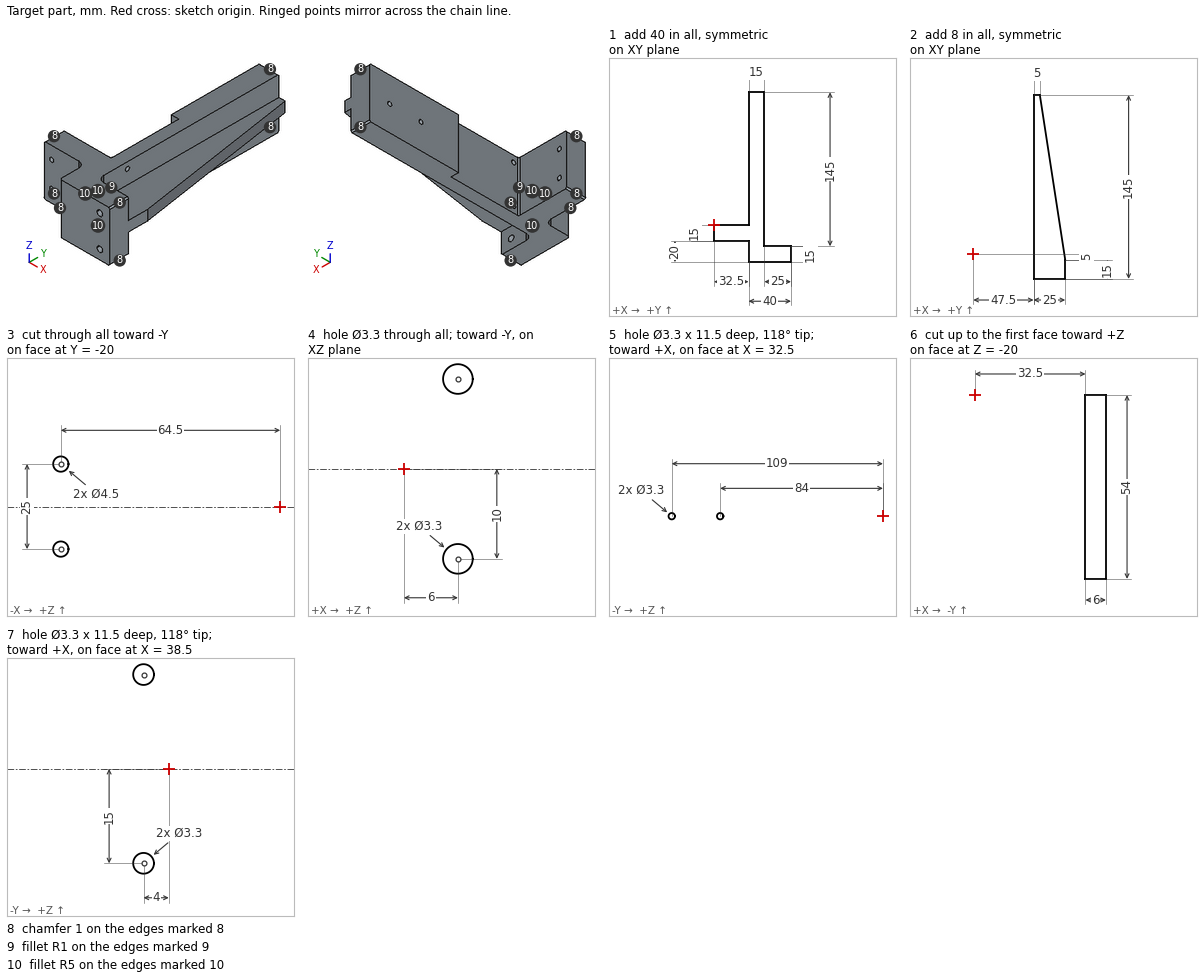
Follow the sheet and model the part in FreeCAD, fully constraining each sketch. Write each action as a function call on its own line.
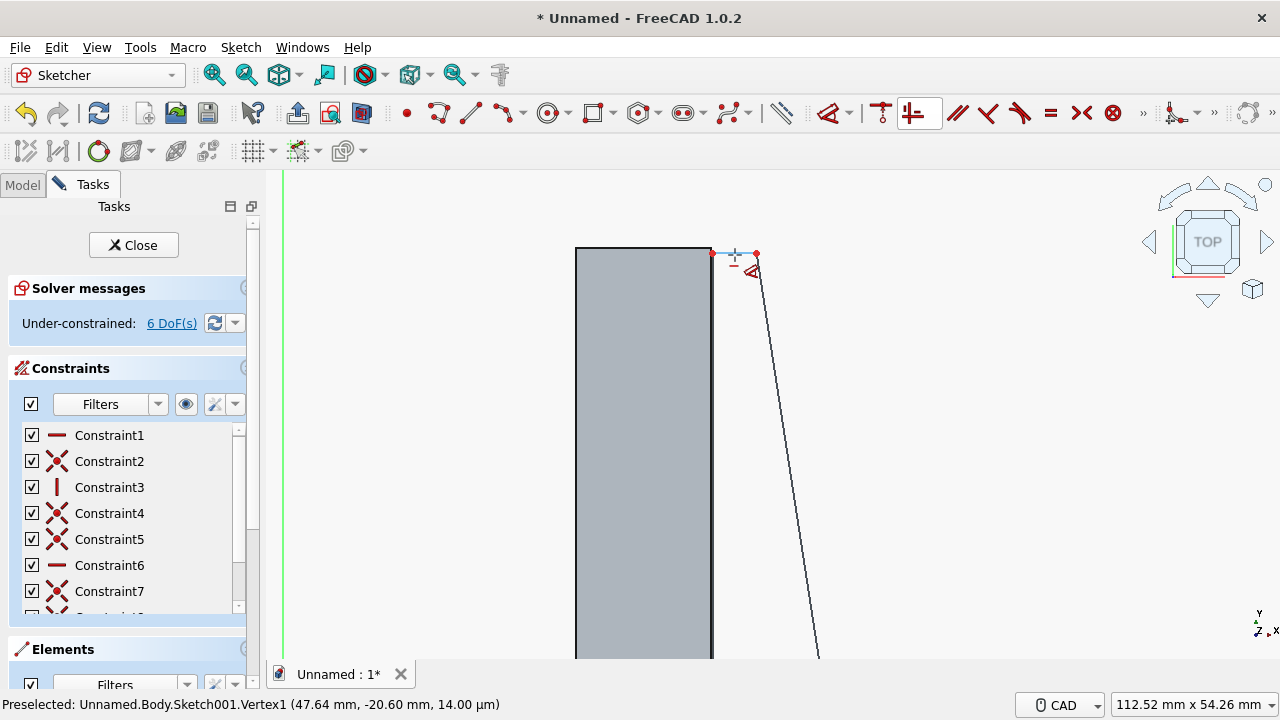
click(735, 253)
click(735, 219)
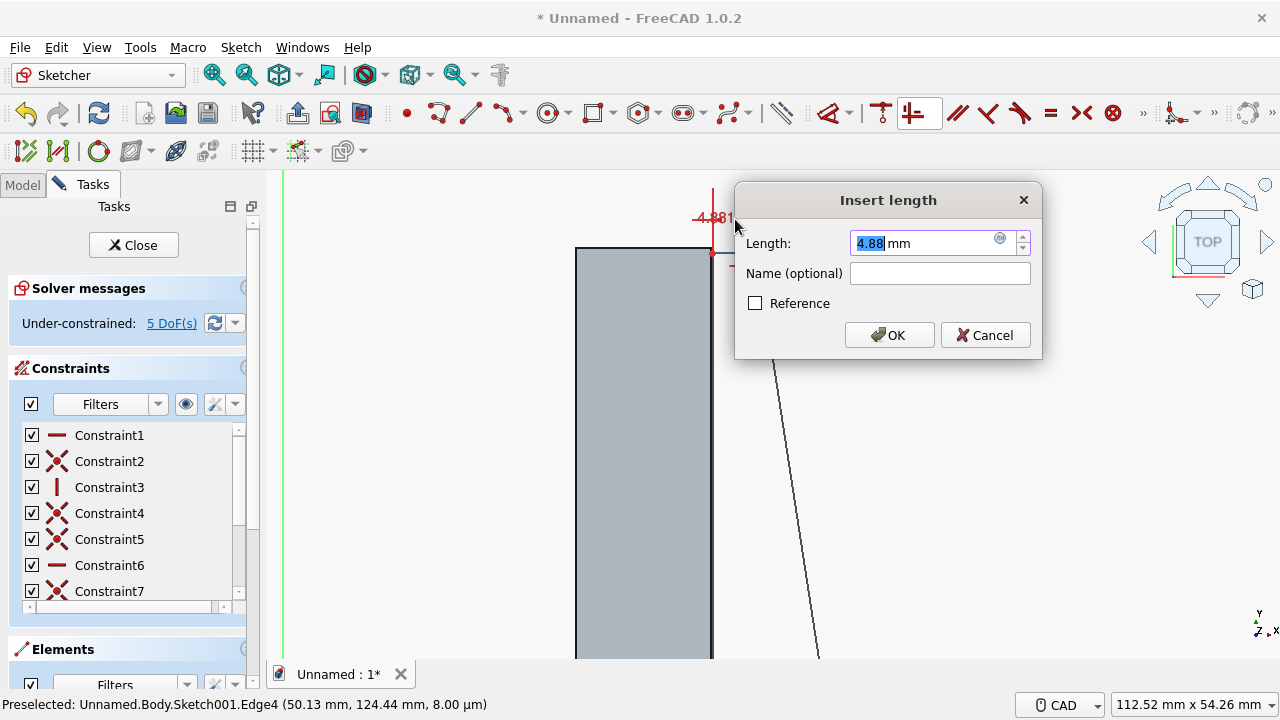
text(5)
key(Return)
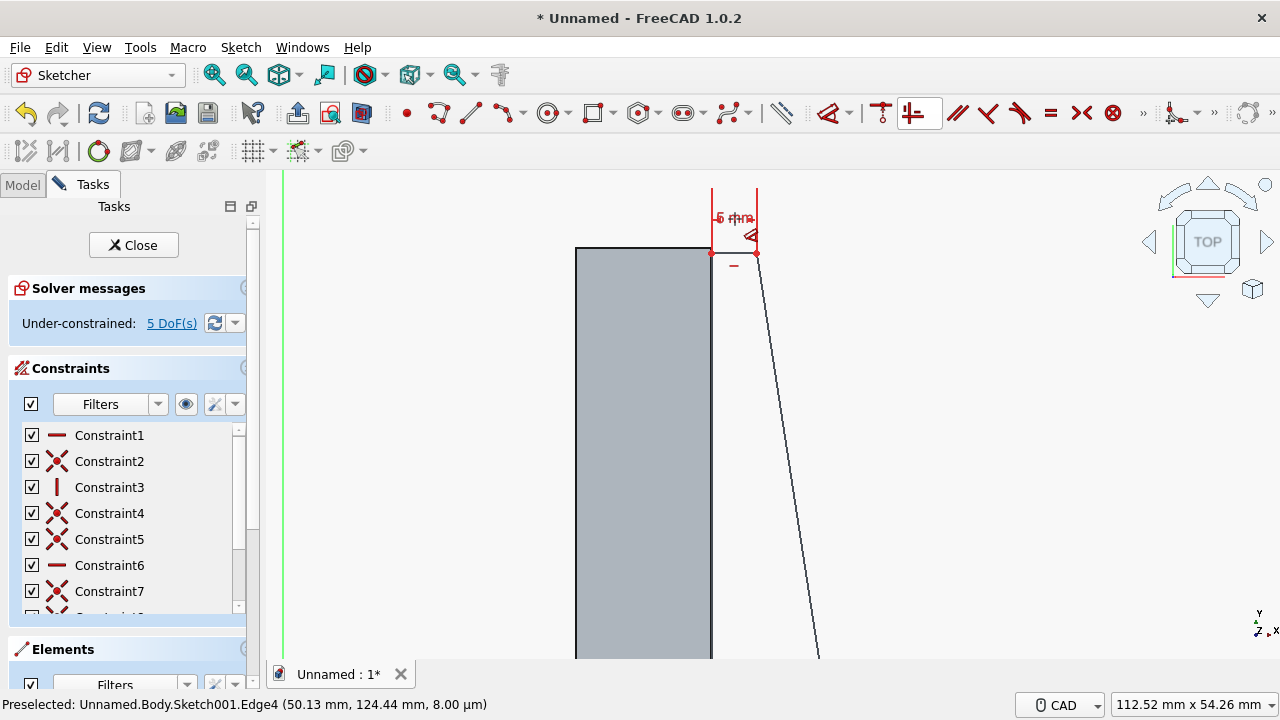
scroll(735, 255, down, 7)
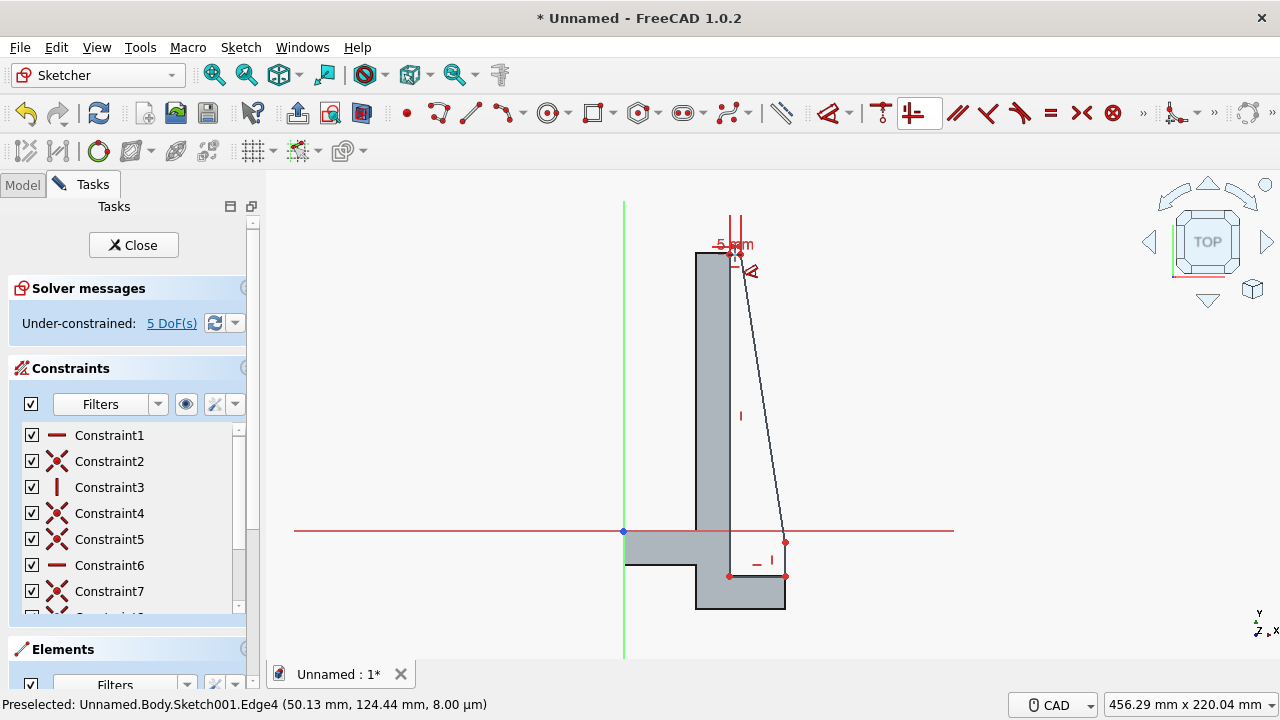
click(746, 577)
click(757, 611)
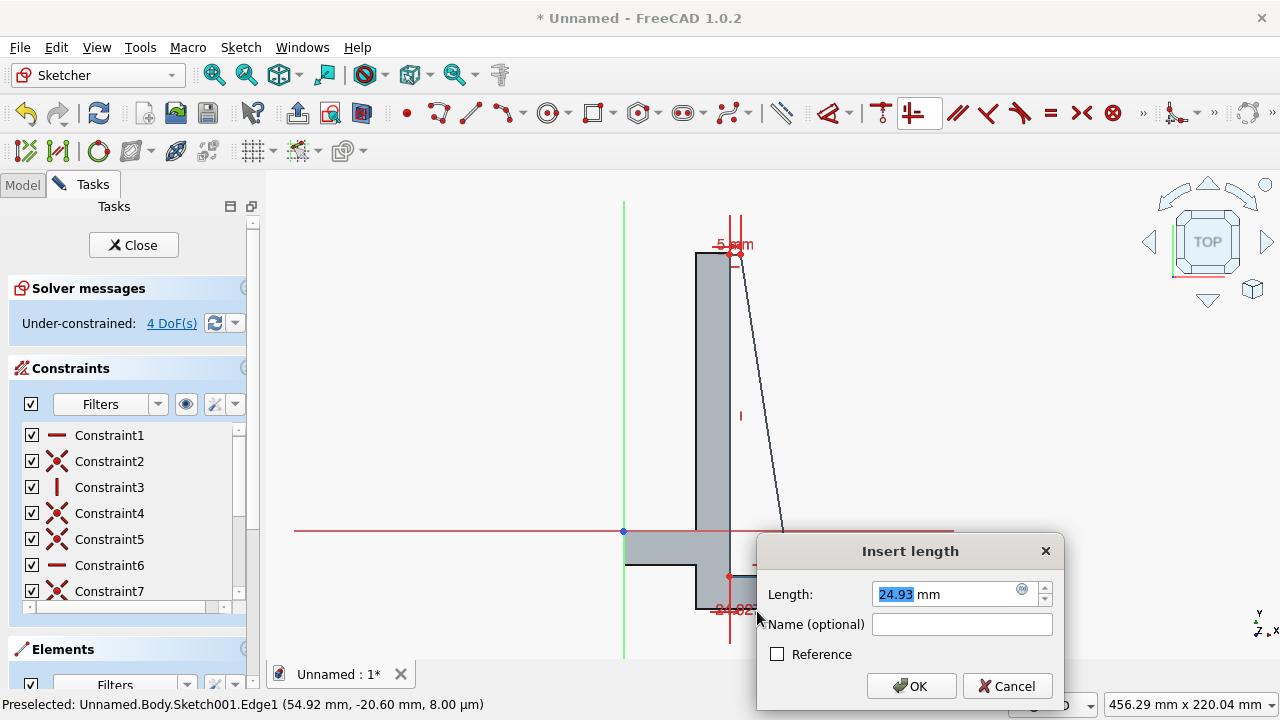
text(25)
key(Return)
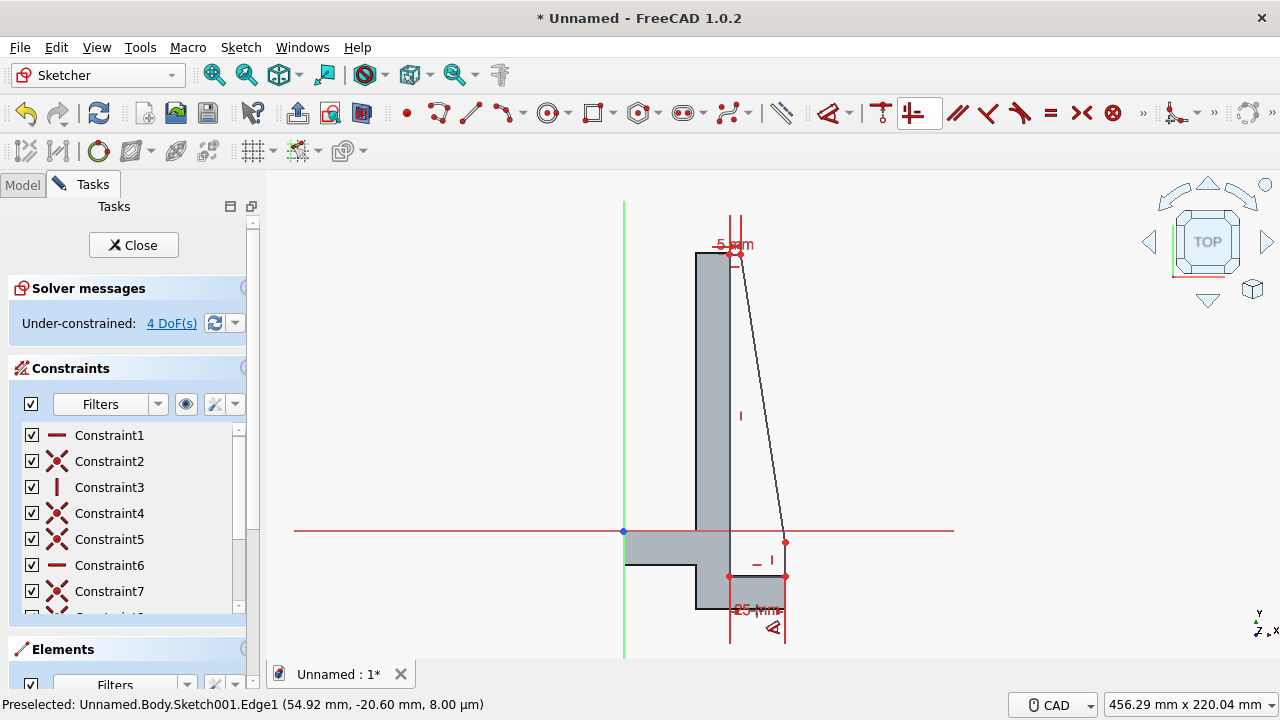
scroll(785, 567, up, 2)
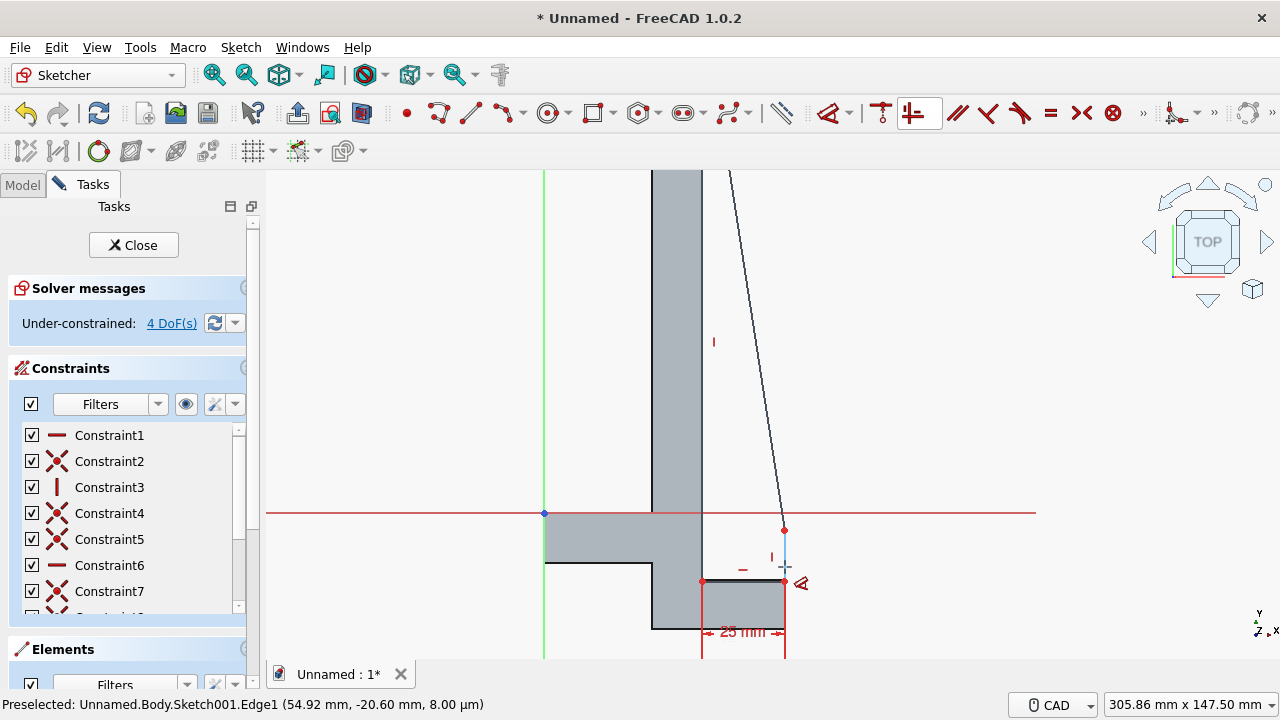
click(785, 566)
click(819, 556)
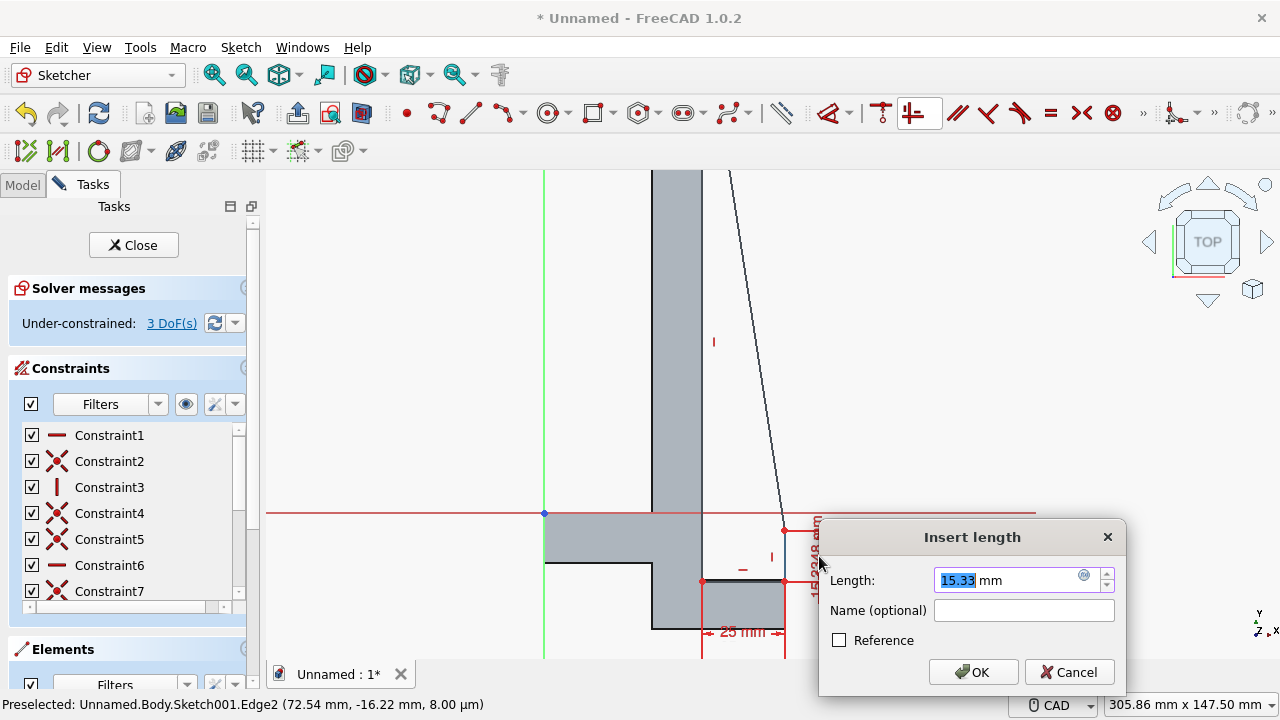
text(15)
key(Return)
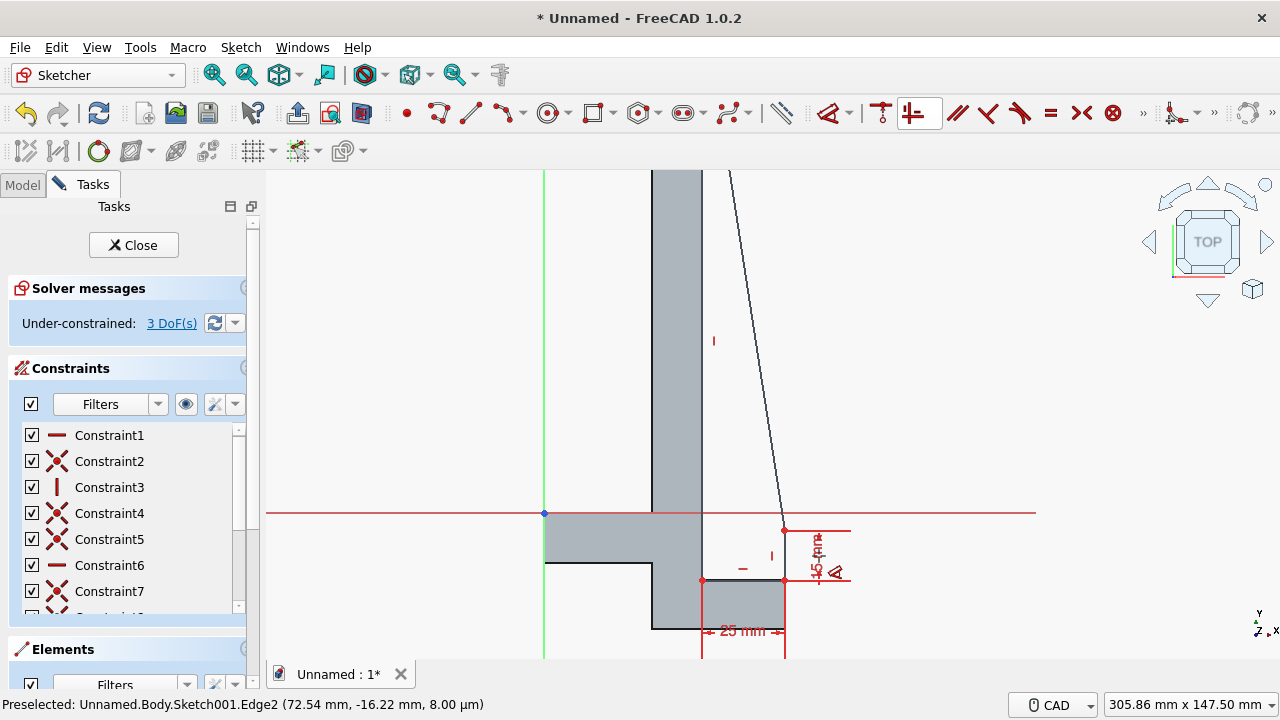
scroll(785, 531, up, 5)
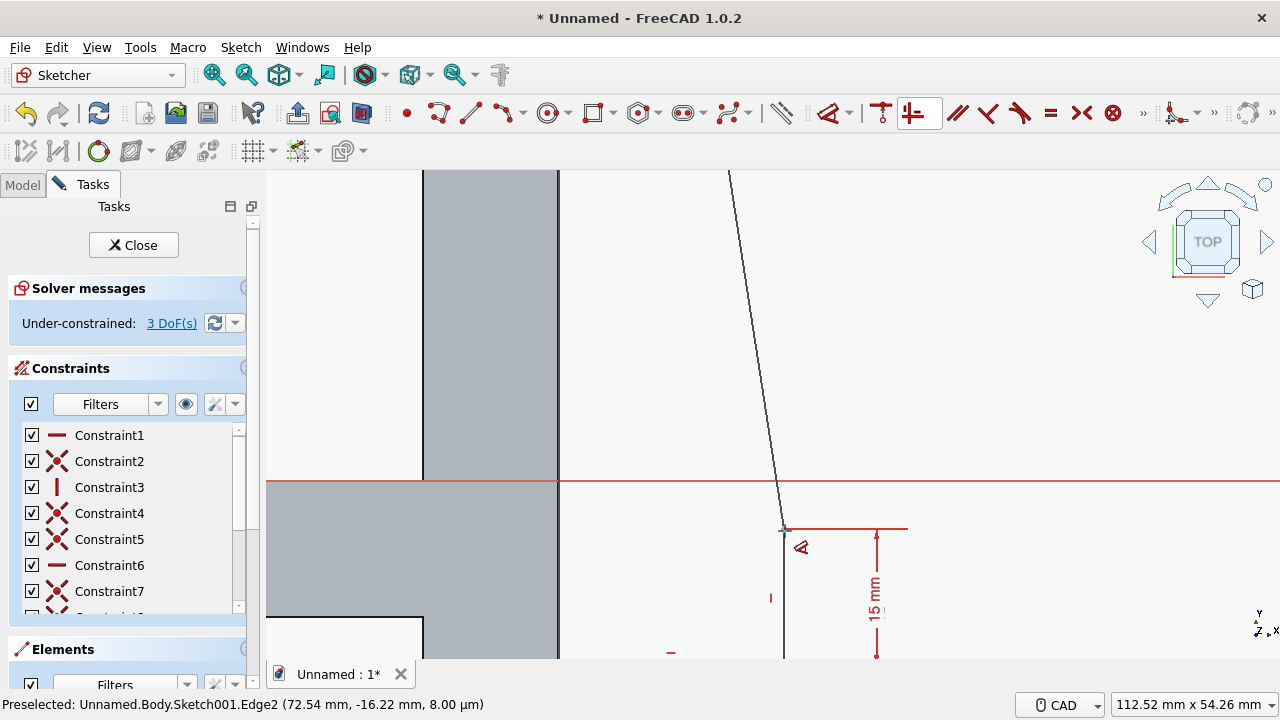
click(784, 529)
click(818, 505)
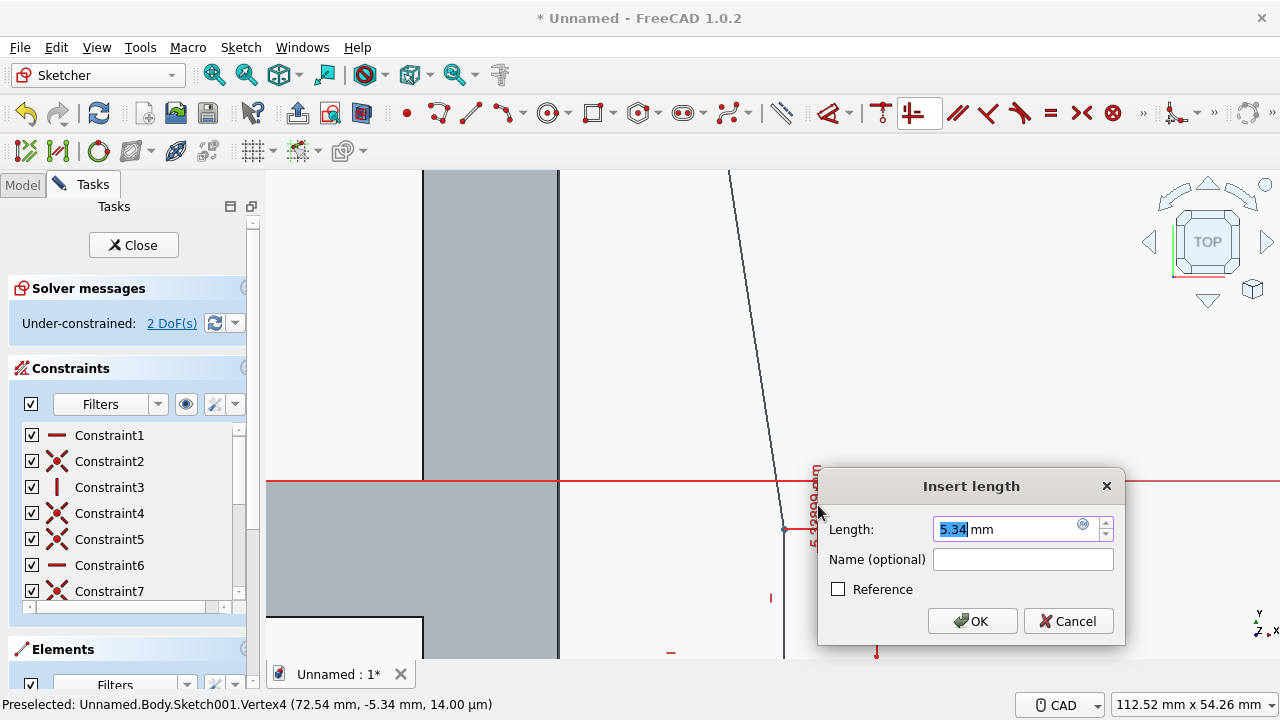
text(5)
key(Return)